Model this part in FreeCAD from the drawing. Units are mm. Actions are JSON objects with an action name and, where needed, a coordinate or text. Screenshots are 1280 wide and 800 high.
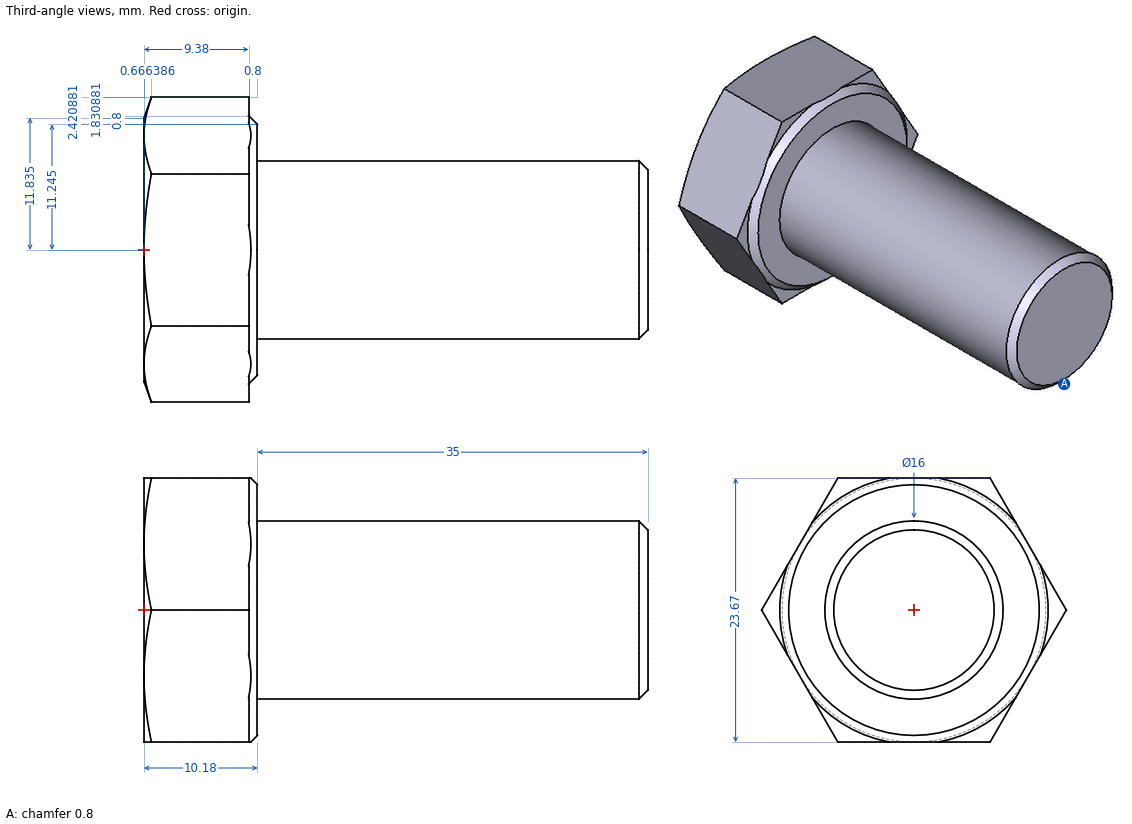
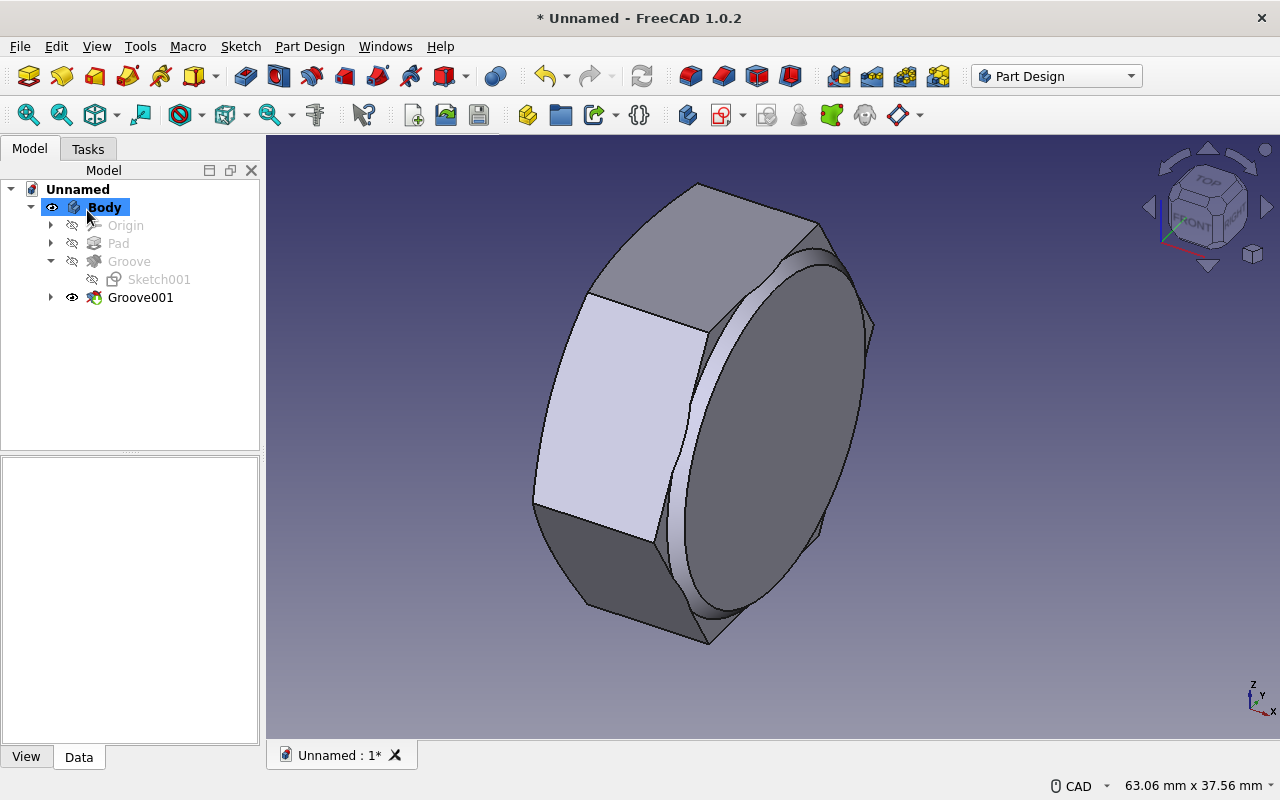
{"action": "left_click", "coordinate": [29, 116]}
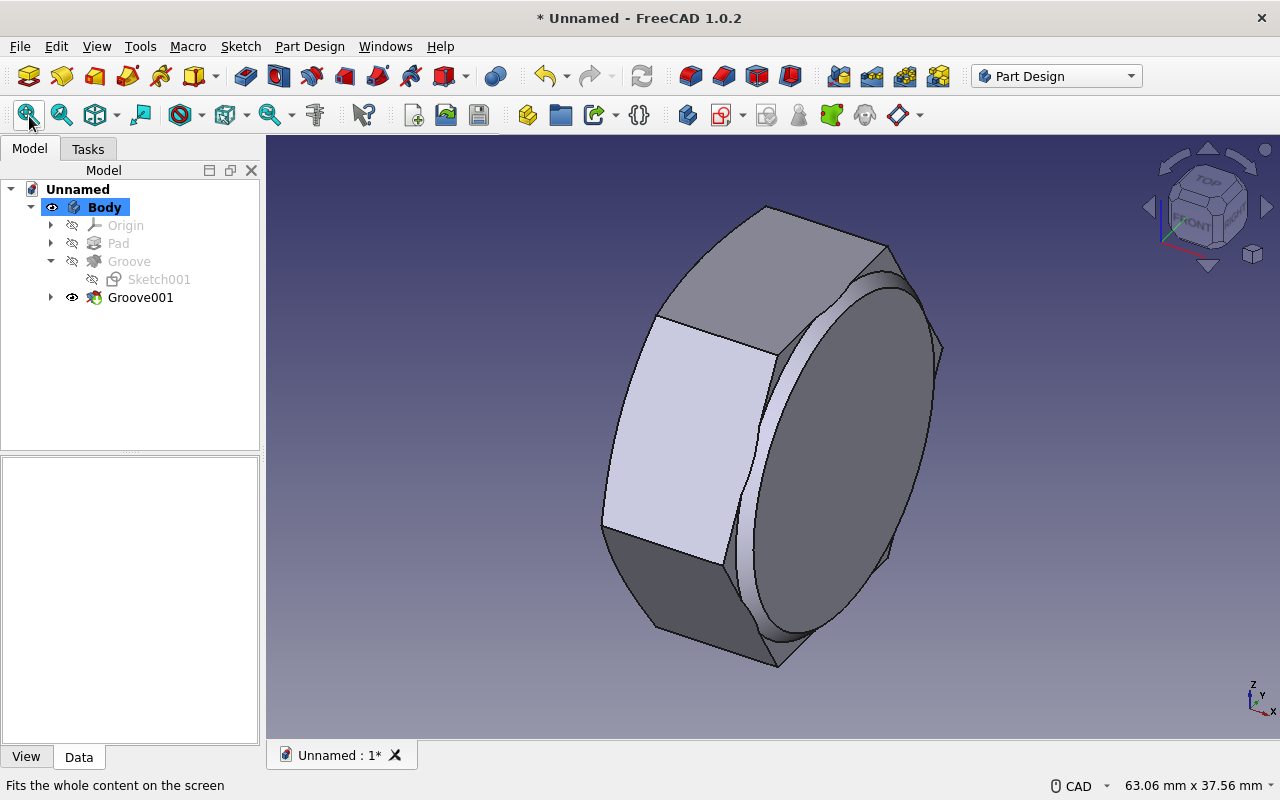
{"action": "left_click", "coordinate": [844, 459]}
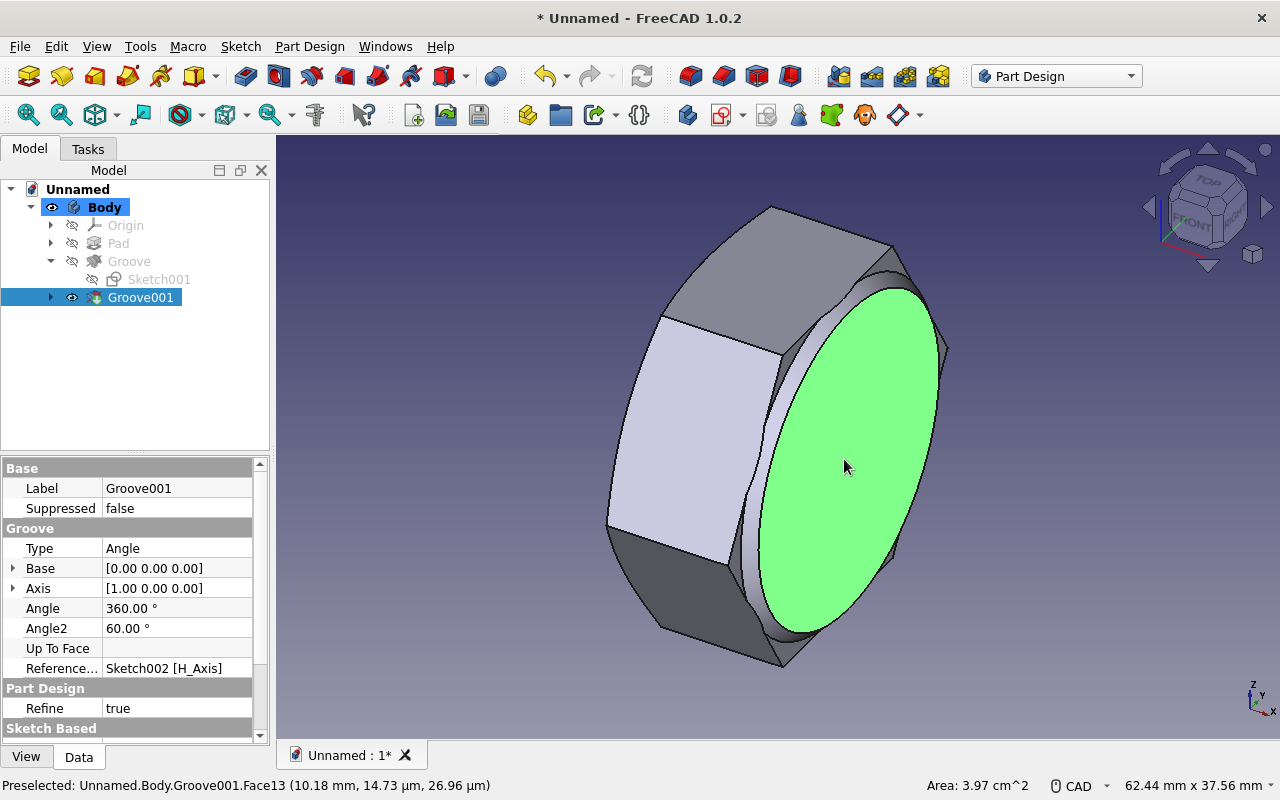
{"action": "left_click", "coordinate": [720, 116]}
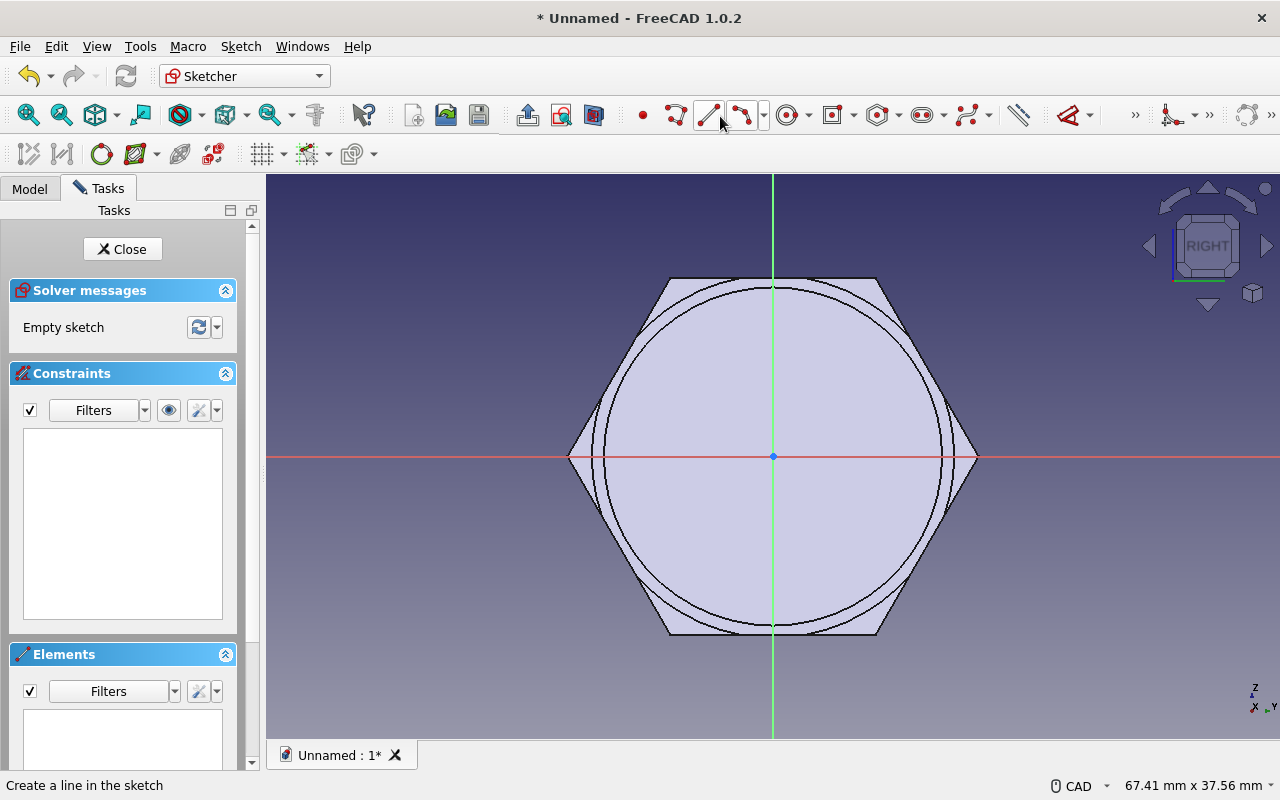
{"action": "scroll", "coordinate": [912, 456], "scroll_direction": "up", "scroll_amount": 2}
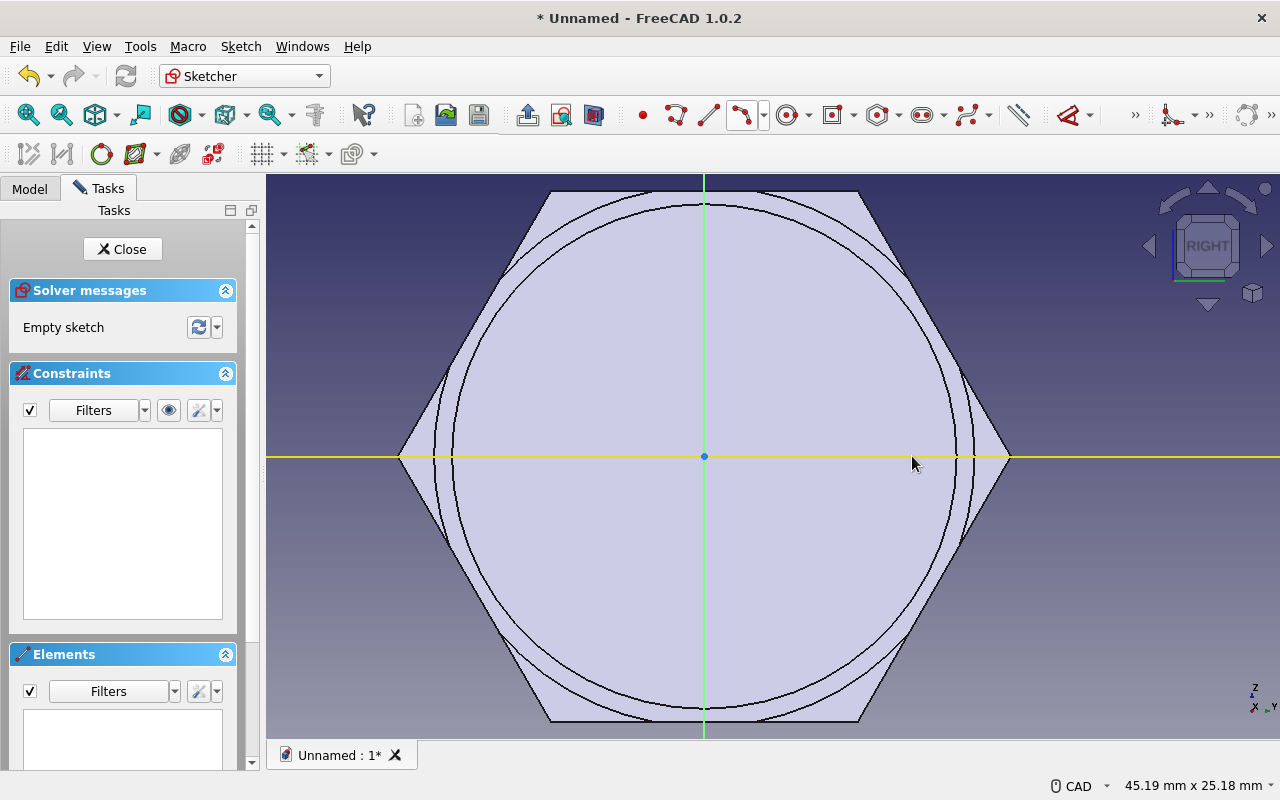
{"action": "key", "text": "g c"}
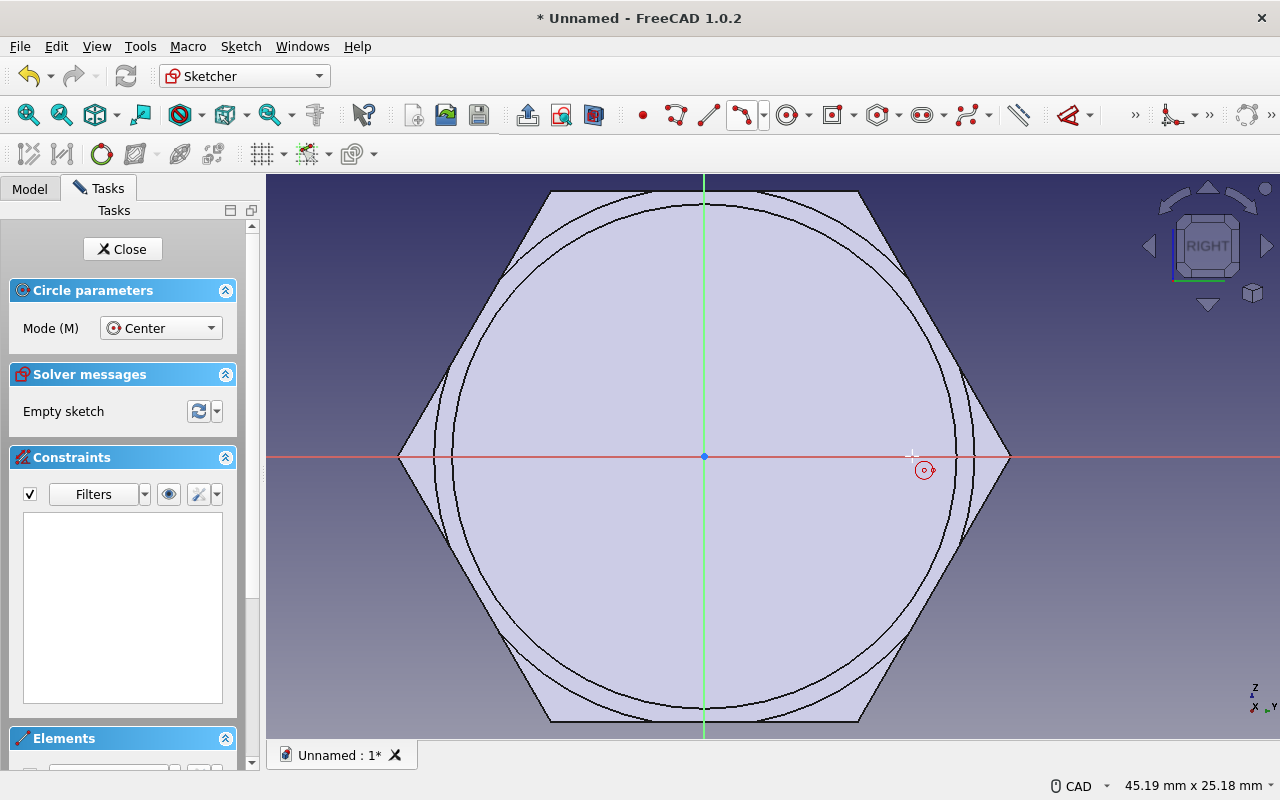
{"action": "left_click", "coordinate": [704, 456]}
{"action": "mouse_move", "coordinate": [831, 330]}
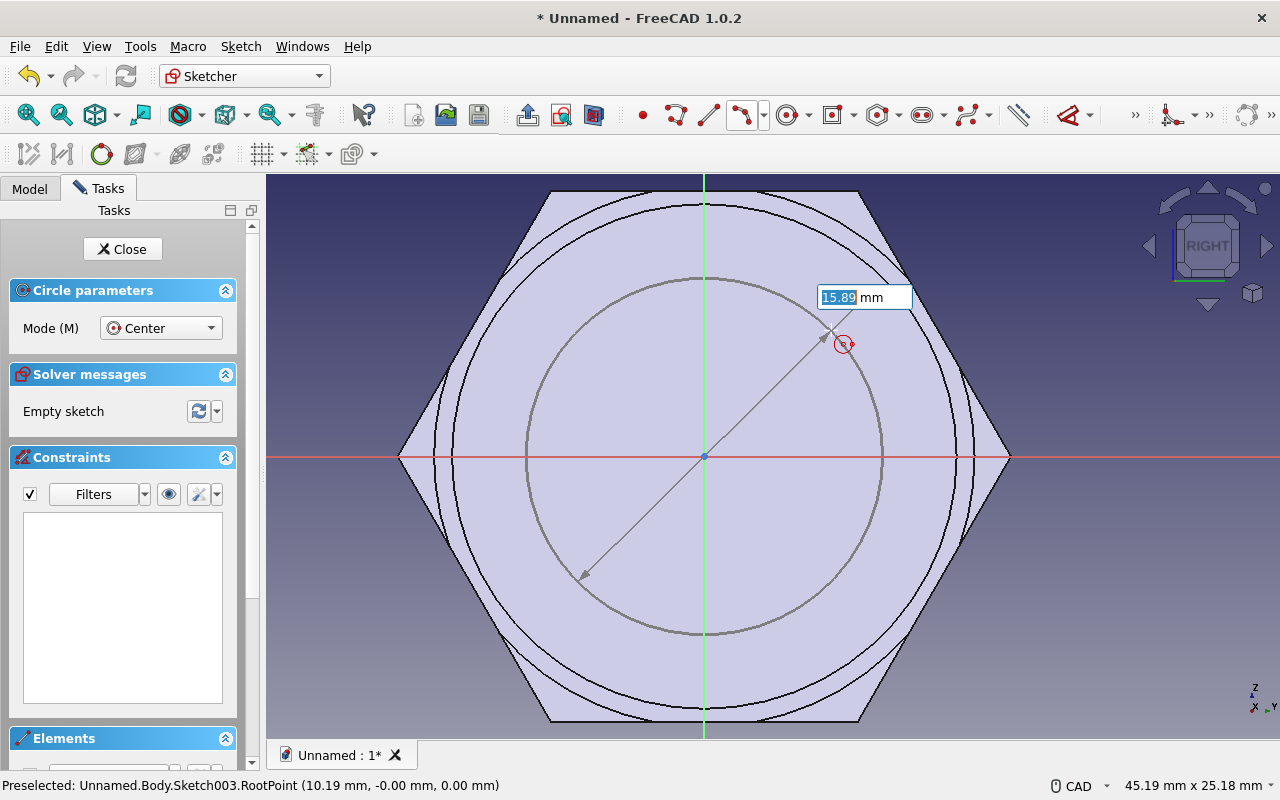
{"action": "type", "text": "16"}
{"action": "key", "text": "Return"}
{"action": "key", "text": "Escape"}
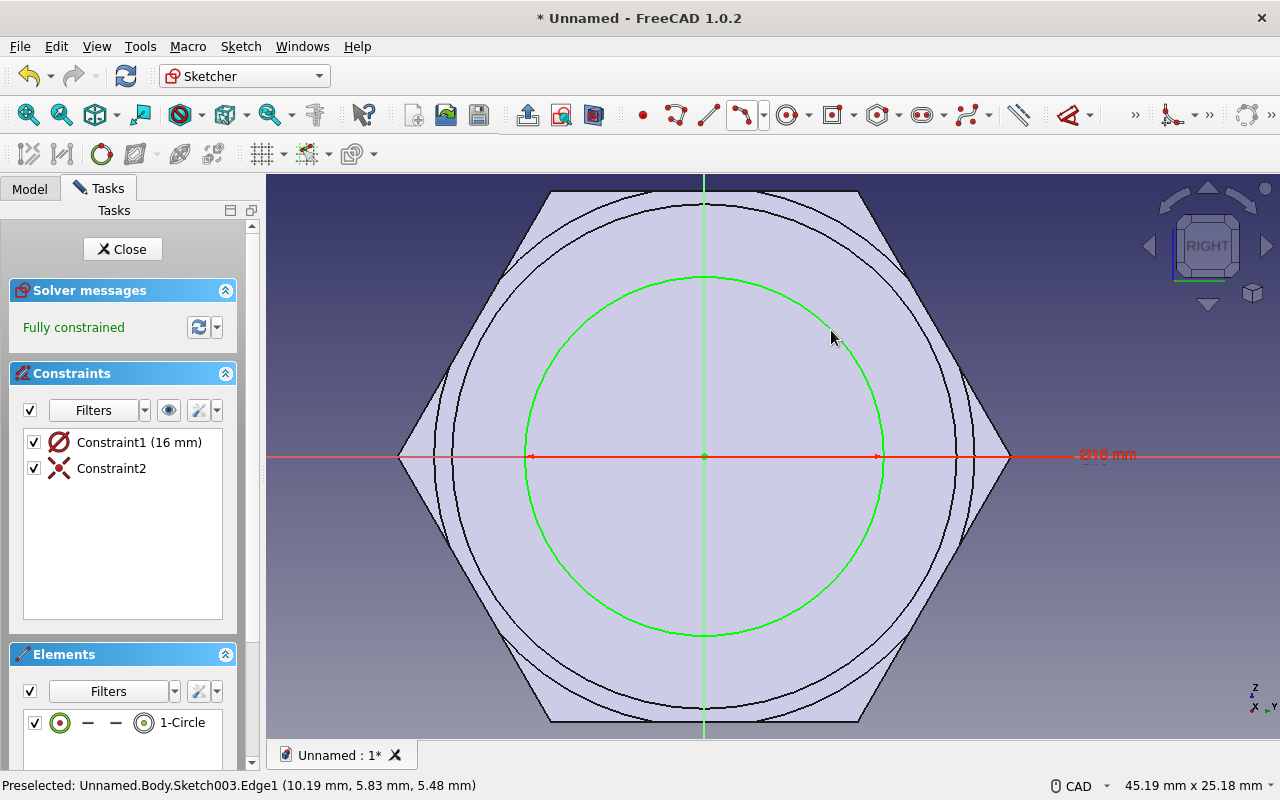
{"action": "left_click", "coordinate": [123, 249]}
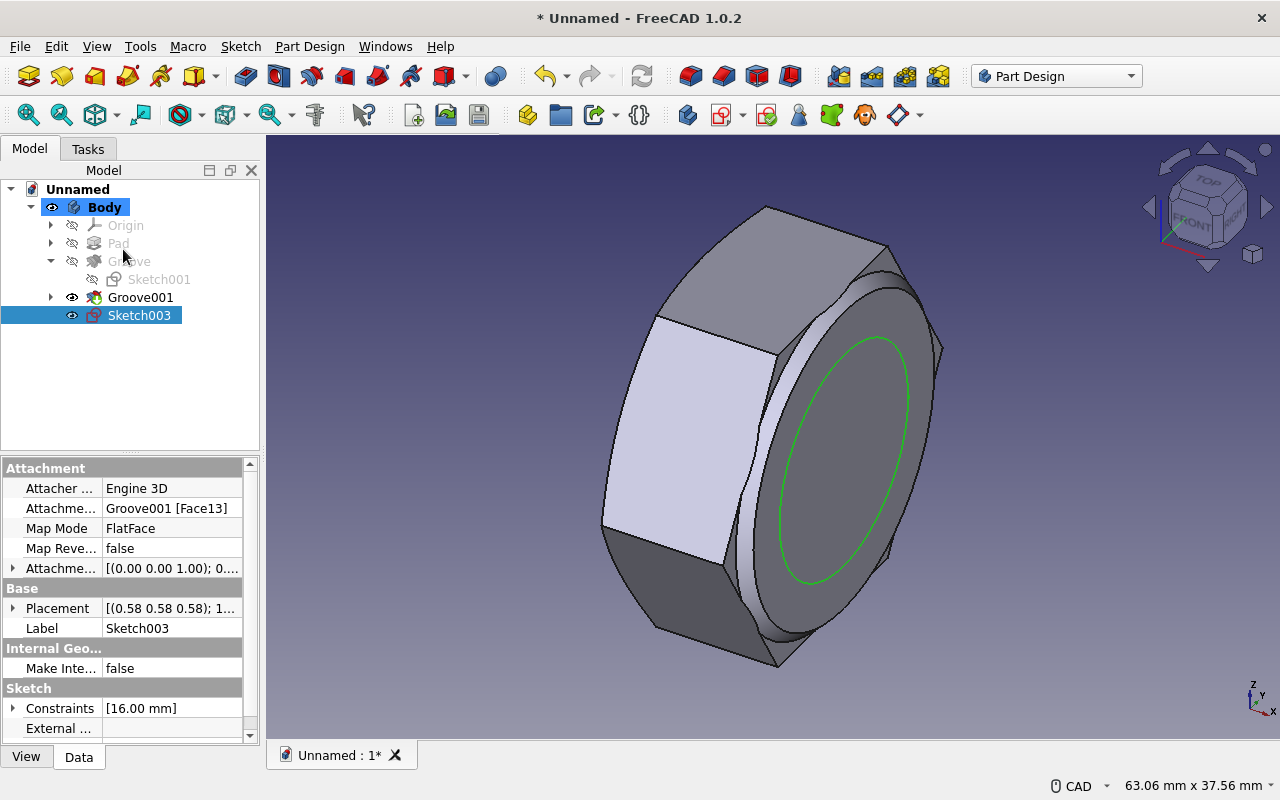
{"action": "left_click", "coordinate": [29, 76]}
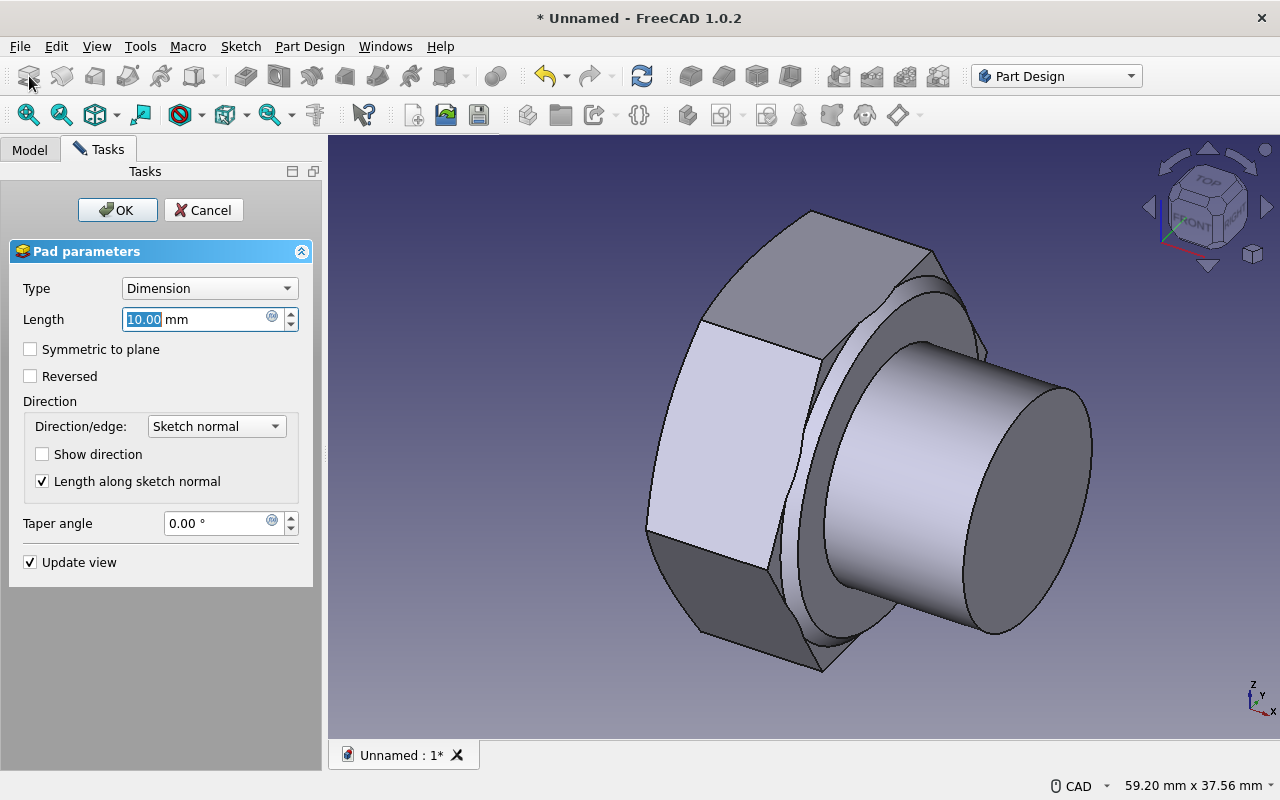
{"action": "type", "text": "35"}
{"action": "key", "text": "Tab"}